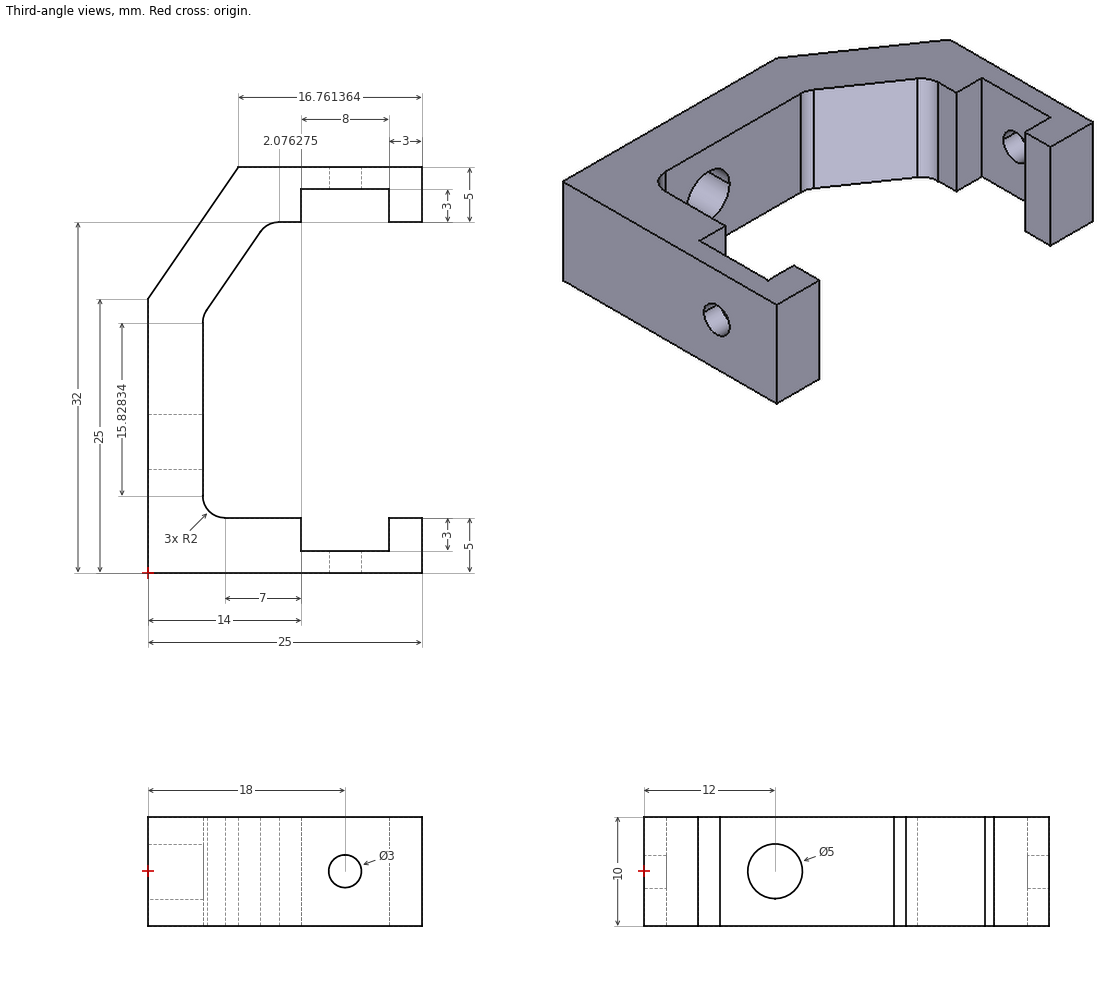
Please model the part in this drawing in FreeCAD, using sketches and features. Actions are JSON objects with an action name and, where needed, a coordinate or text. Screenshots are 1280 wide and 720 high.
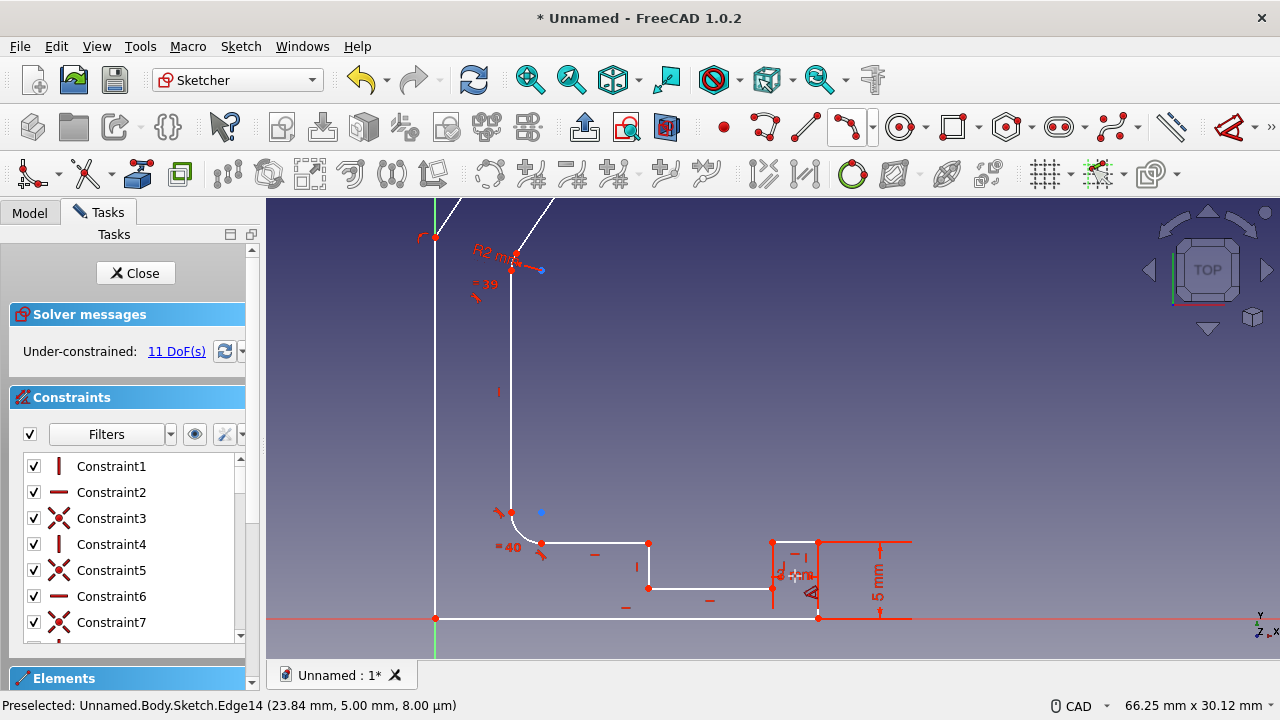
{"action": "left_click", "coordinate": [773, 556]}
{"action": "left_click", "coordinate": [739, 555]}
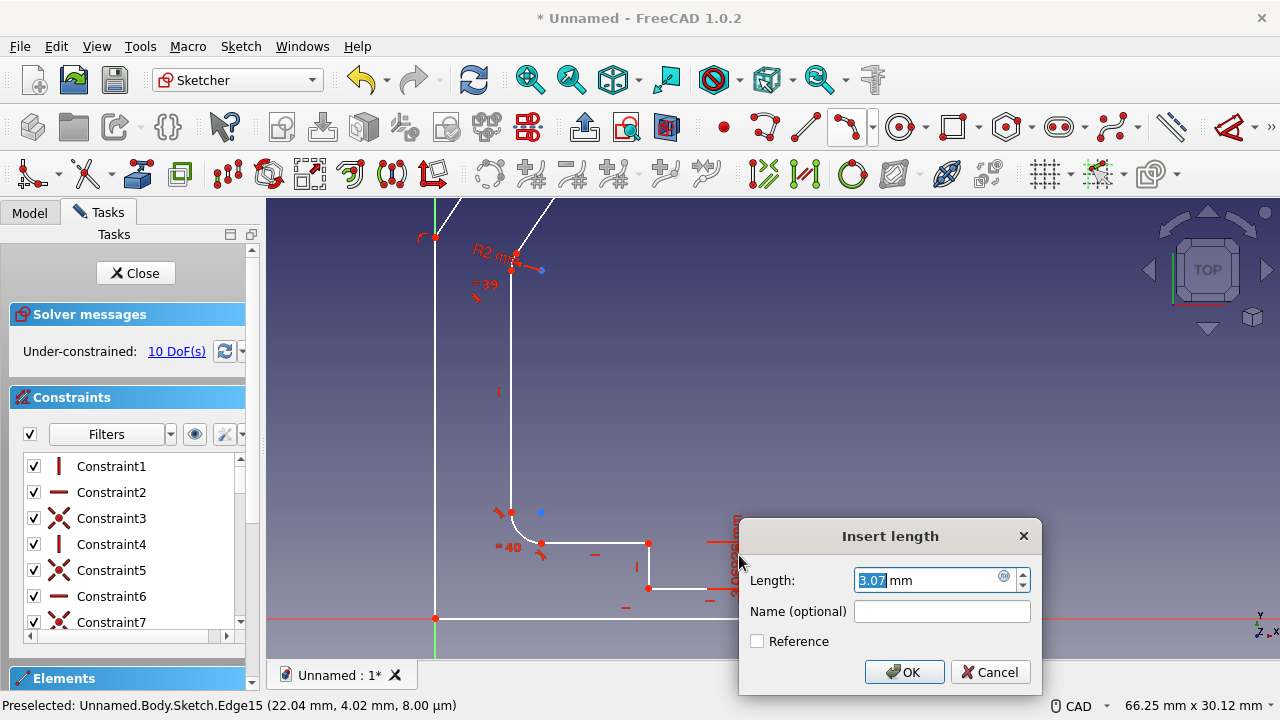
{"action": "type", "text": "3"}
{"action": "key", "text": "Return"}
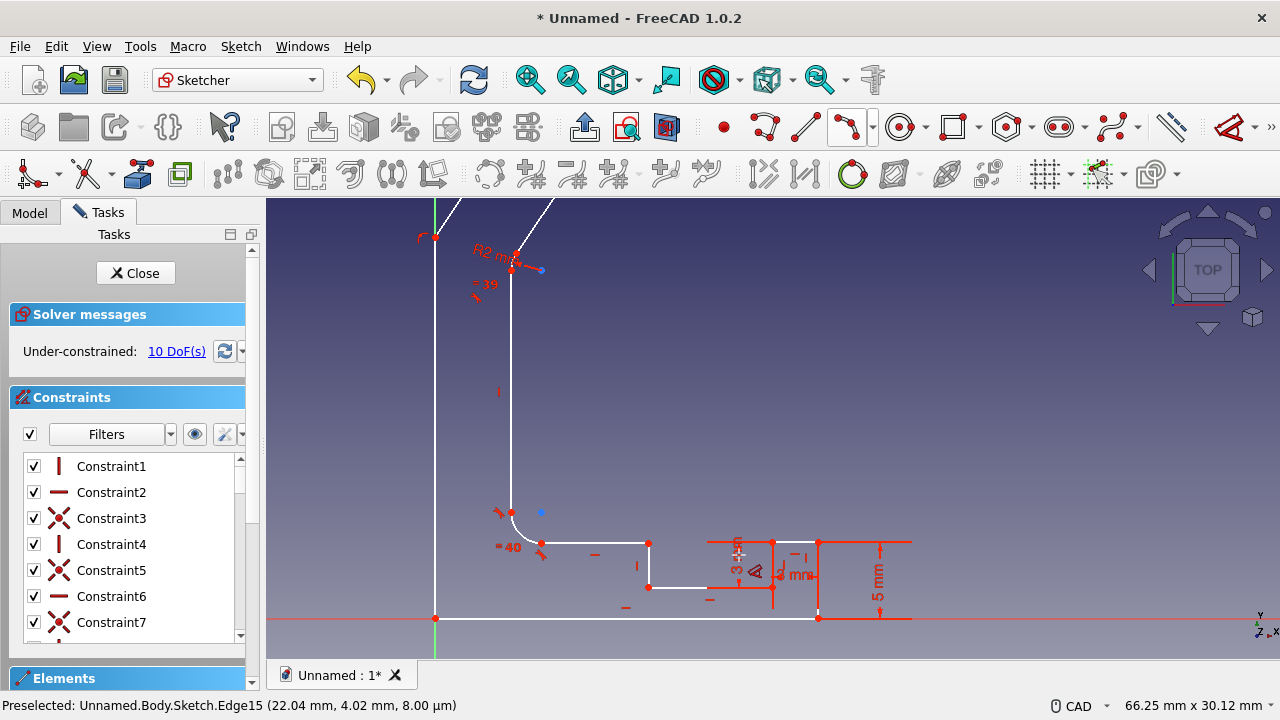
{"action": "left_click", "coordinate": [735, 588]}
{"action": "left_click", "coordinate": [667, 554]}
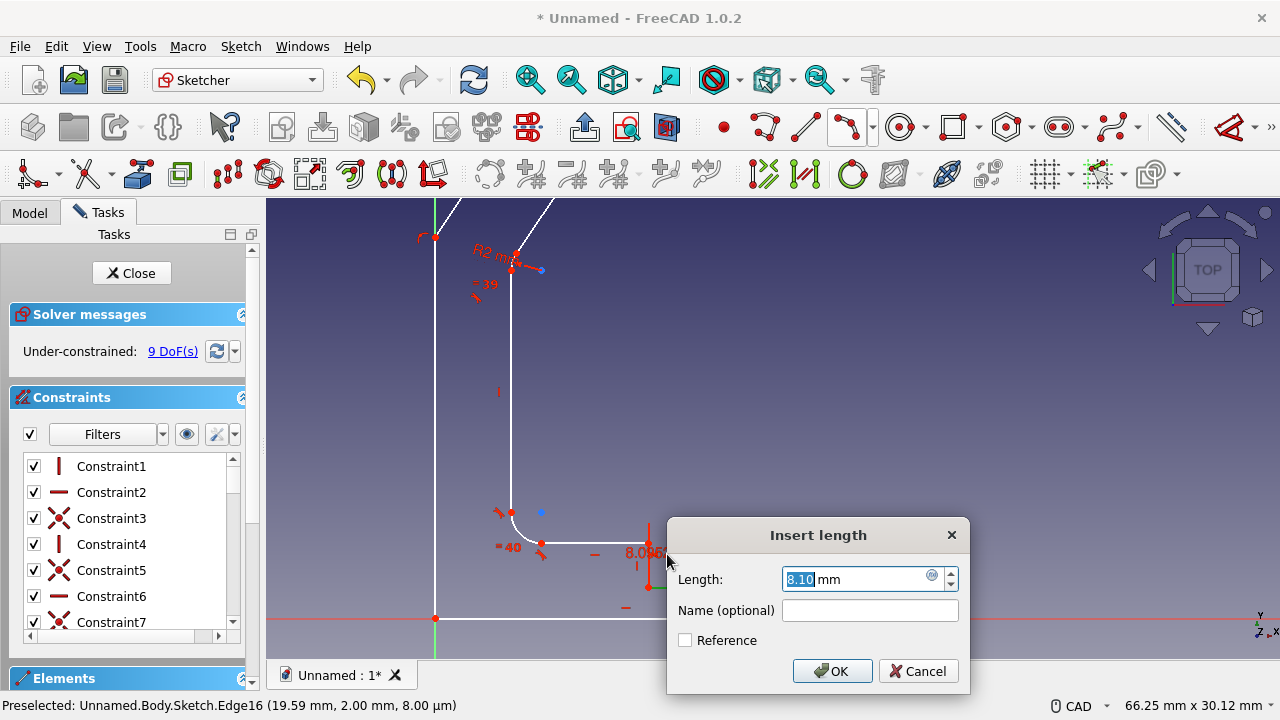
{"action": "type", "text": "8"}
{"action": "key", "text": "Return"}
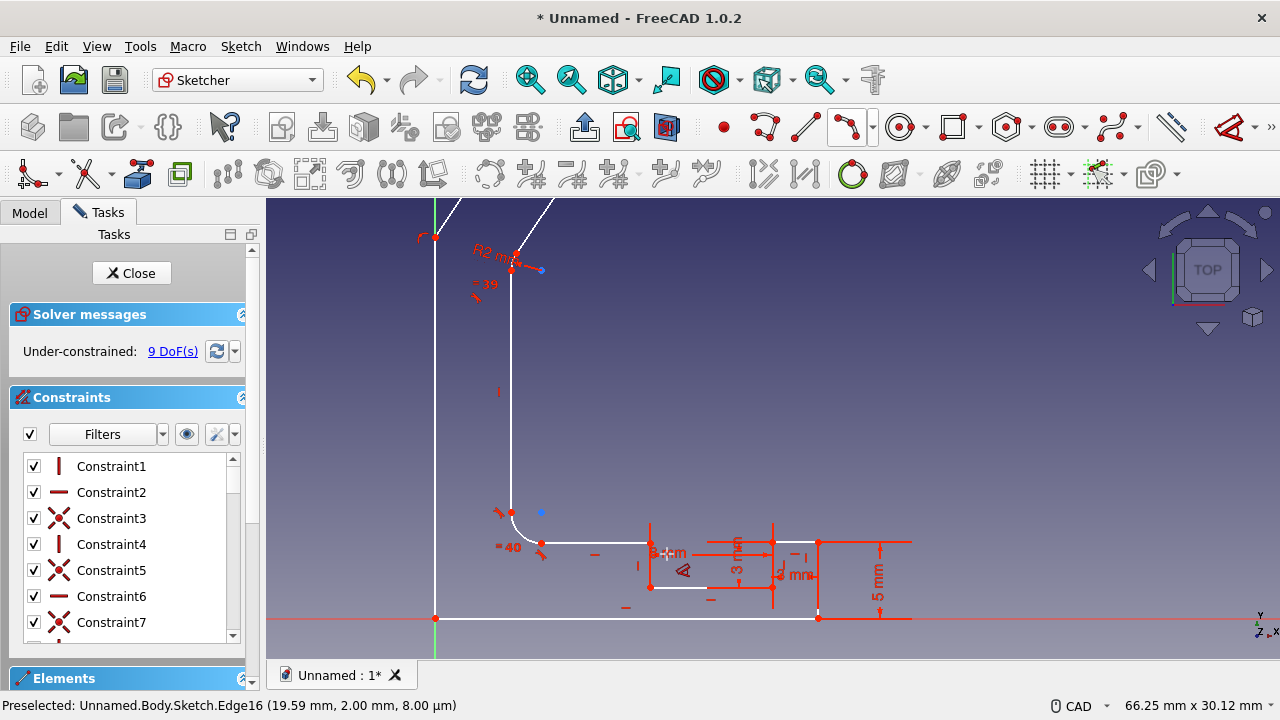
{"action": "left_click", "coordinate": [650, 575]}
{"action": "left_click", "coordinate": [616, 576]}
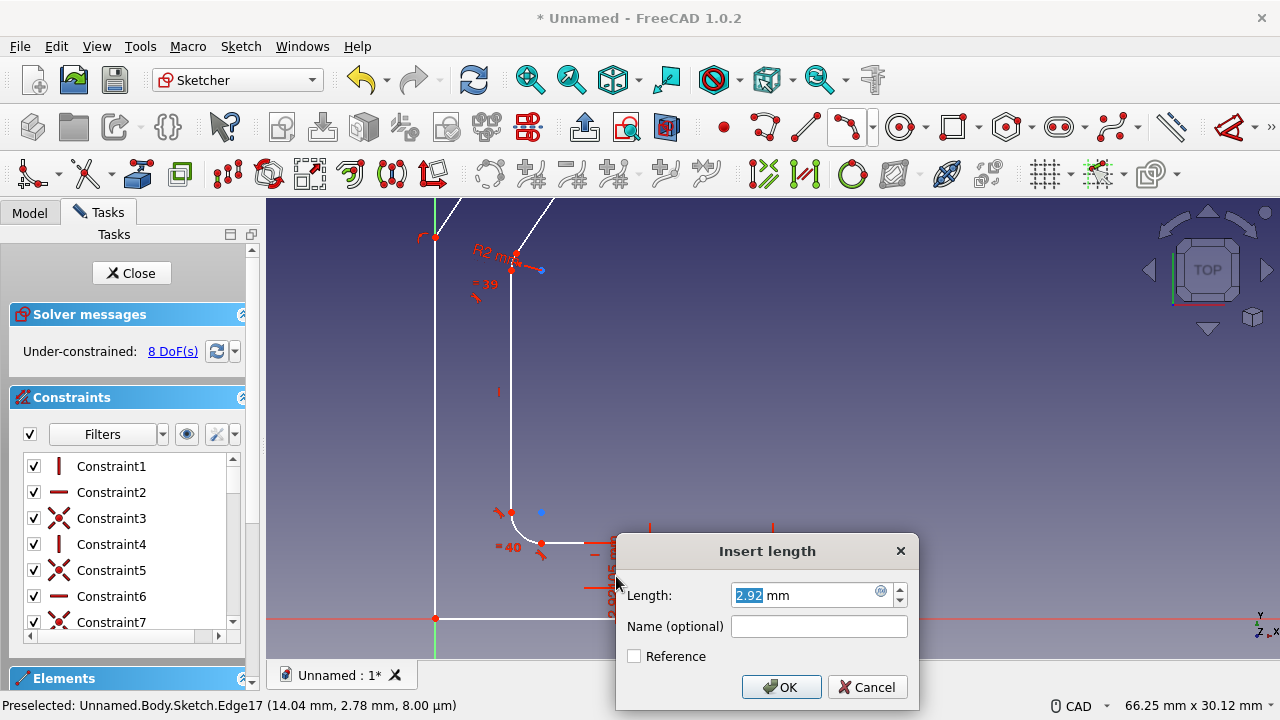
{"action": "type", "text": "3"}
{"action": "key", "text": "Return"}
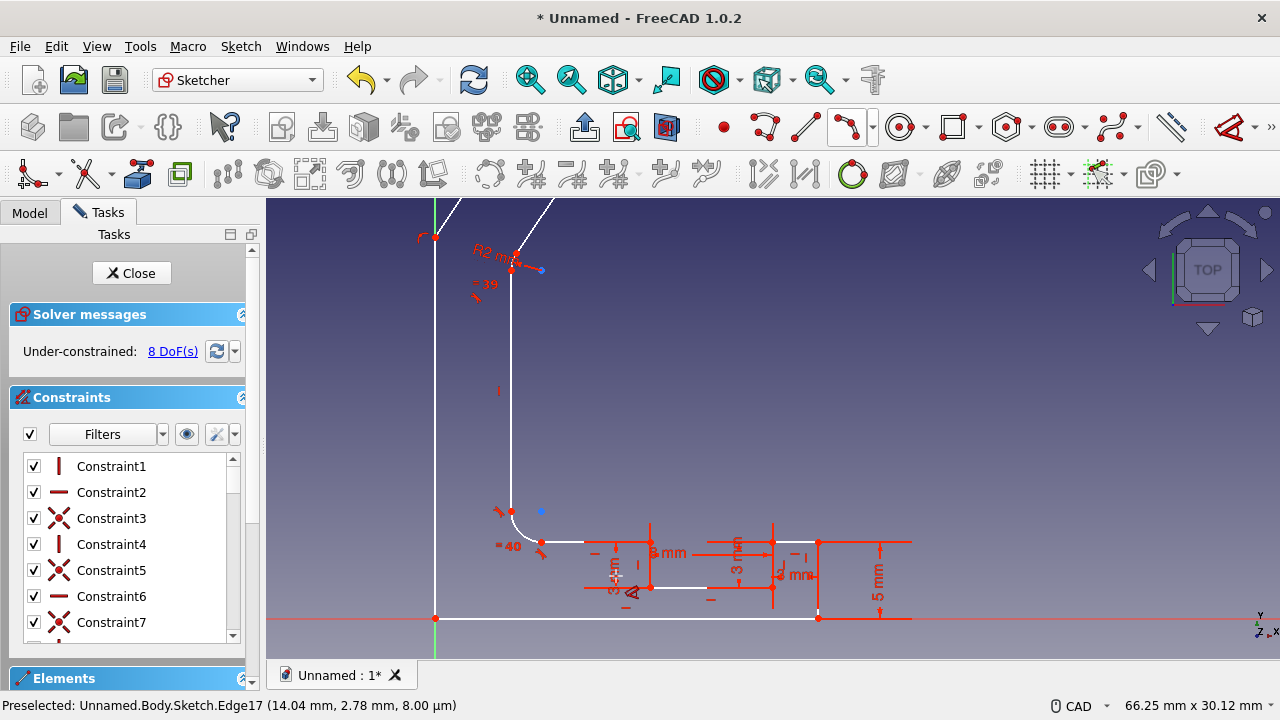
{"action": "left_click", "coordinate": [618, 542]}
{"action": "left_click", "coordinate": [596, 508]}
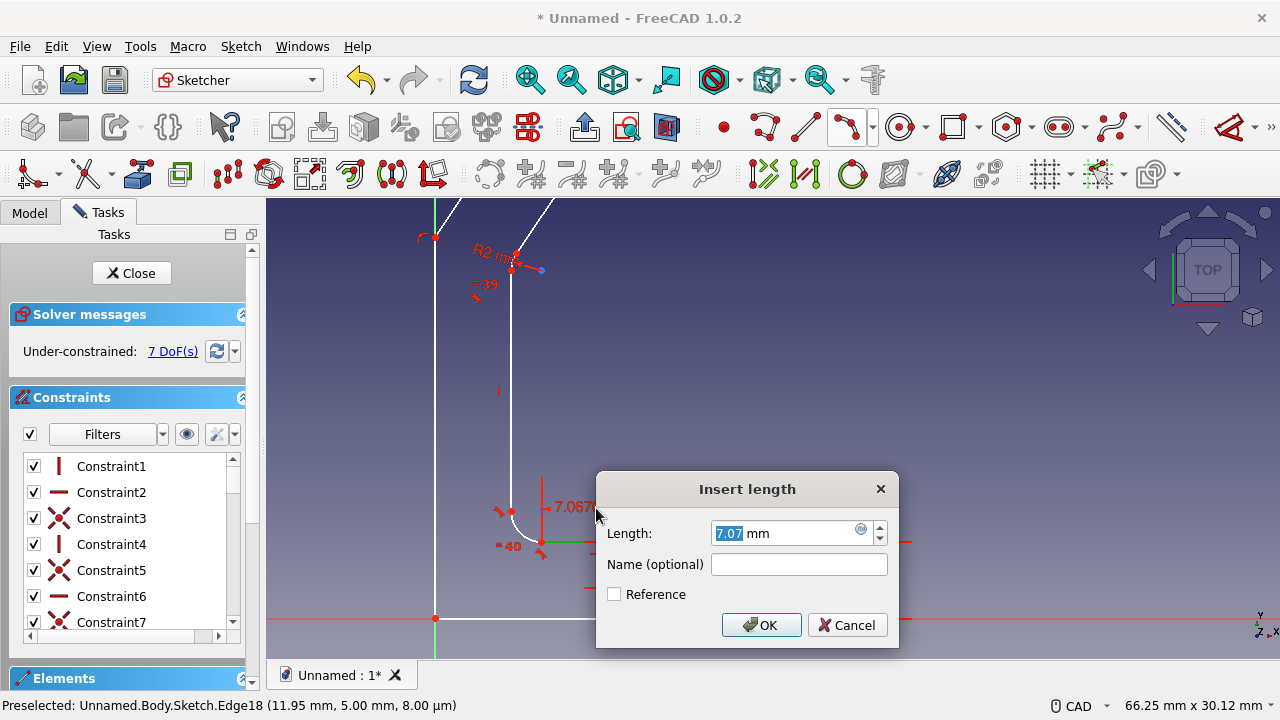
{"action": "type", "text": "7"}
{"action": "key", "text": "Return"}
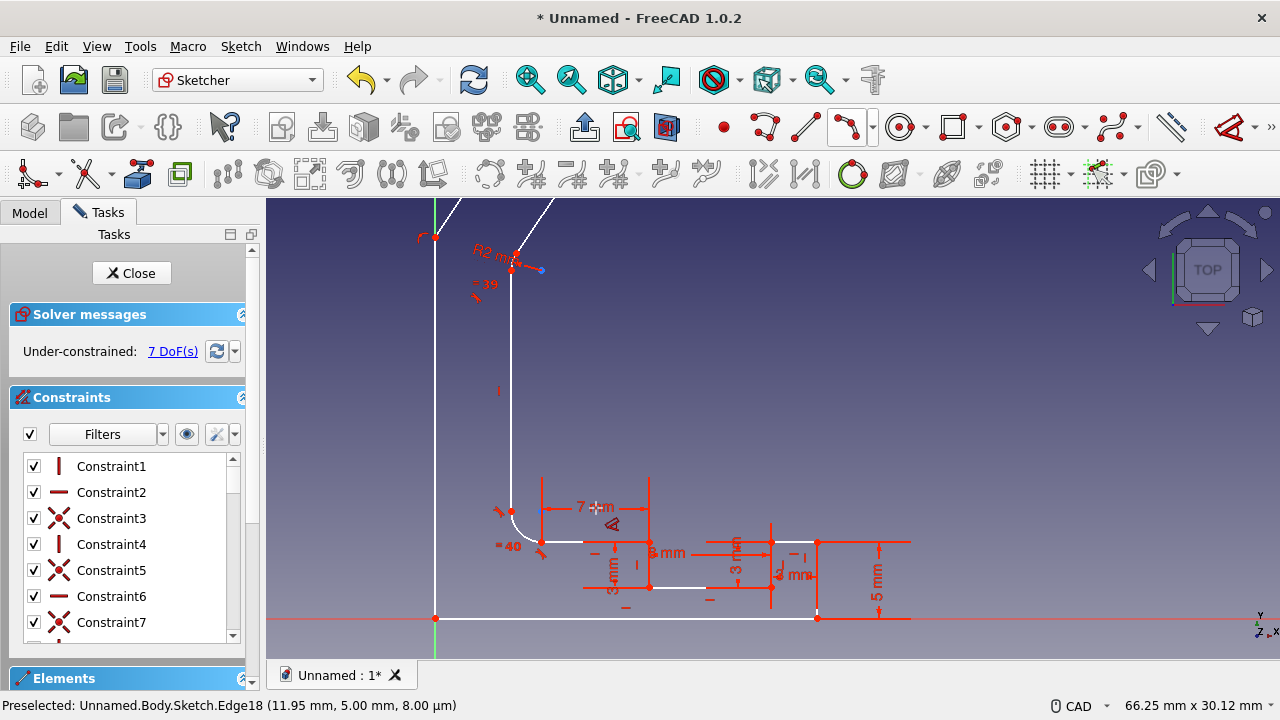
{"action": "left_click", "coordinate": [435, 352]}
{"action": "left_click", "coordinate": [401, 428]}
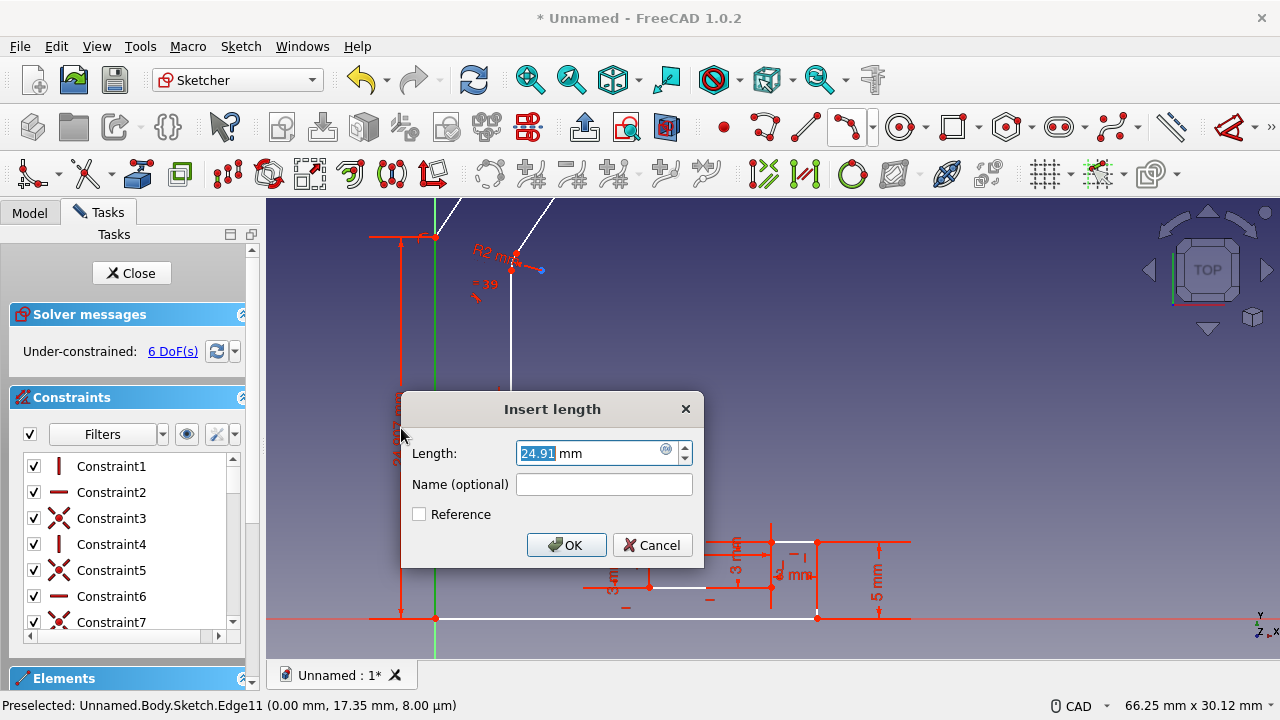
{"action": "type", "text": "25"}
{"action": "key", "text": "Return"}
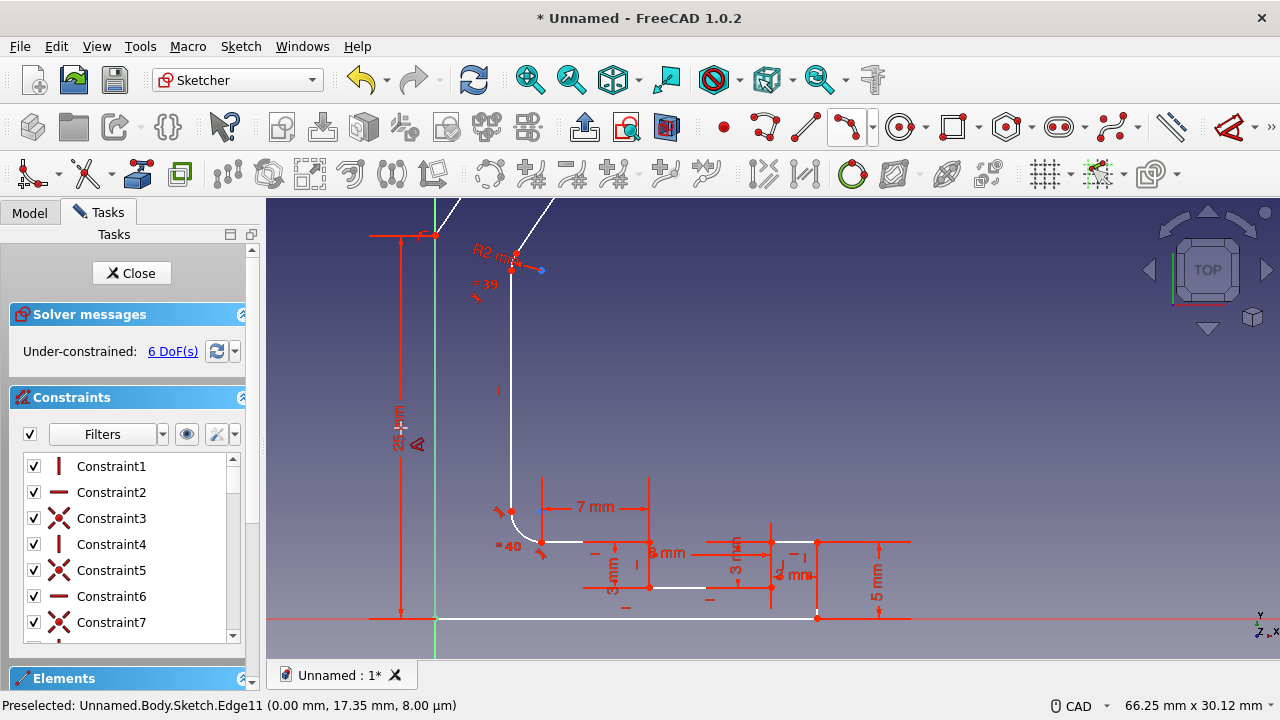
{"action": "left_click", "coordinate": [550, 619]}
{"action": "left_click", "coordinate": [538, 585]}